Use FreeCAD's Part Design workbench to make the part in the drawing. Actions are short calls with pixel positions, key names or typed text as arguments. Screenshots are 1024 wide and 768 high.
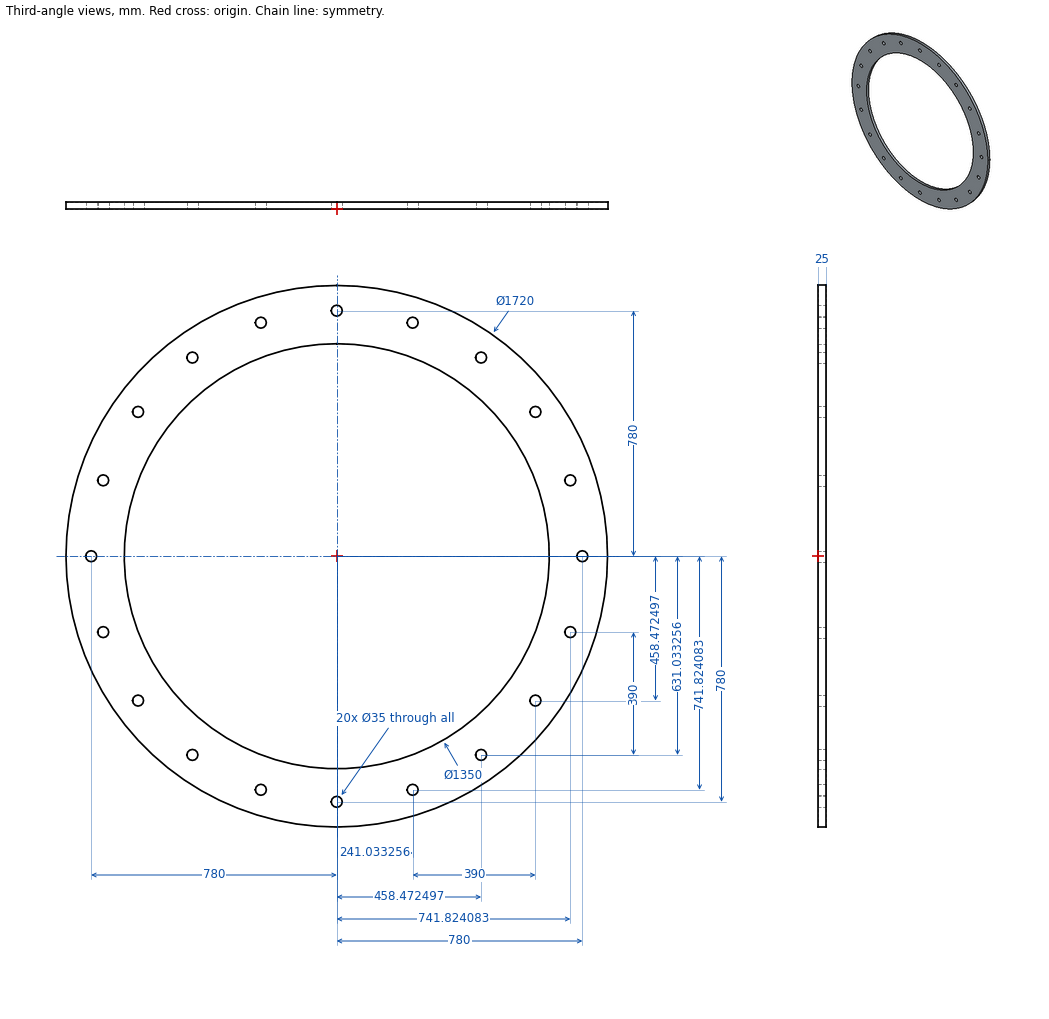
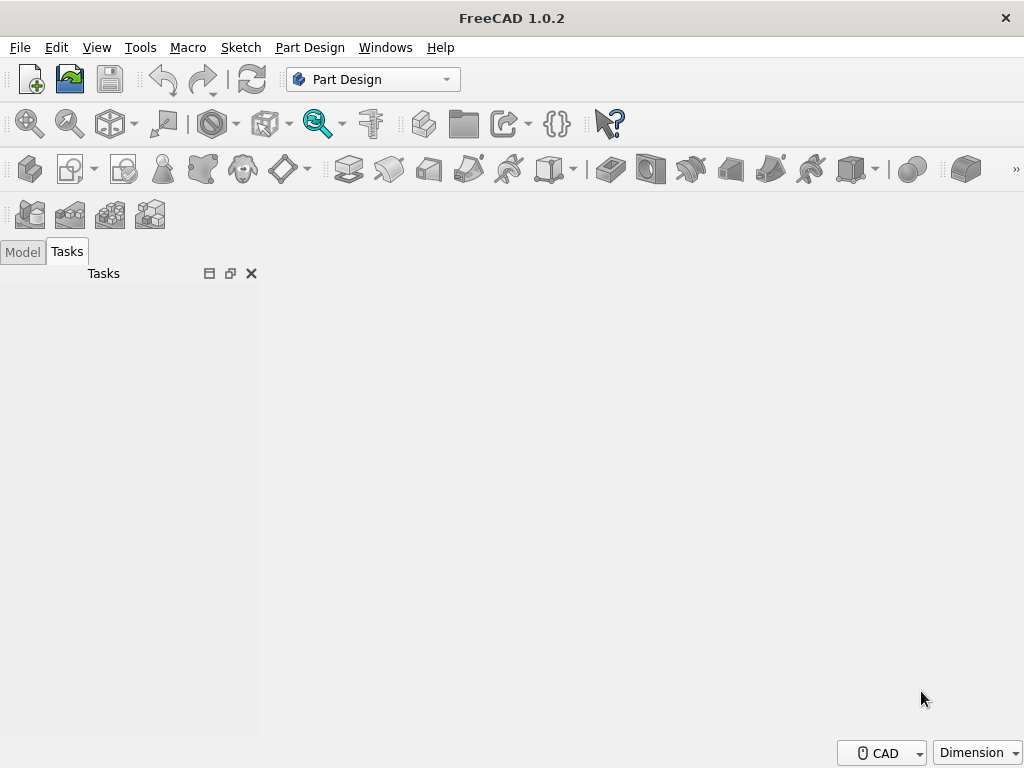
key(ctrl+n)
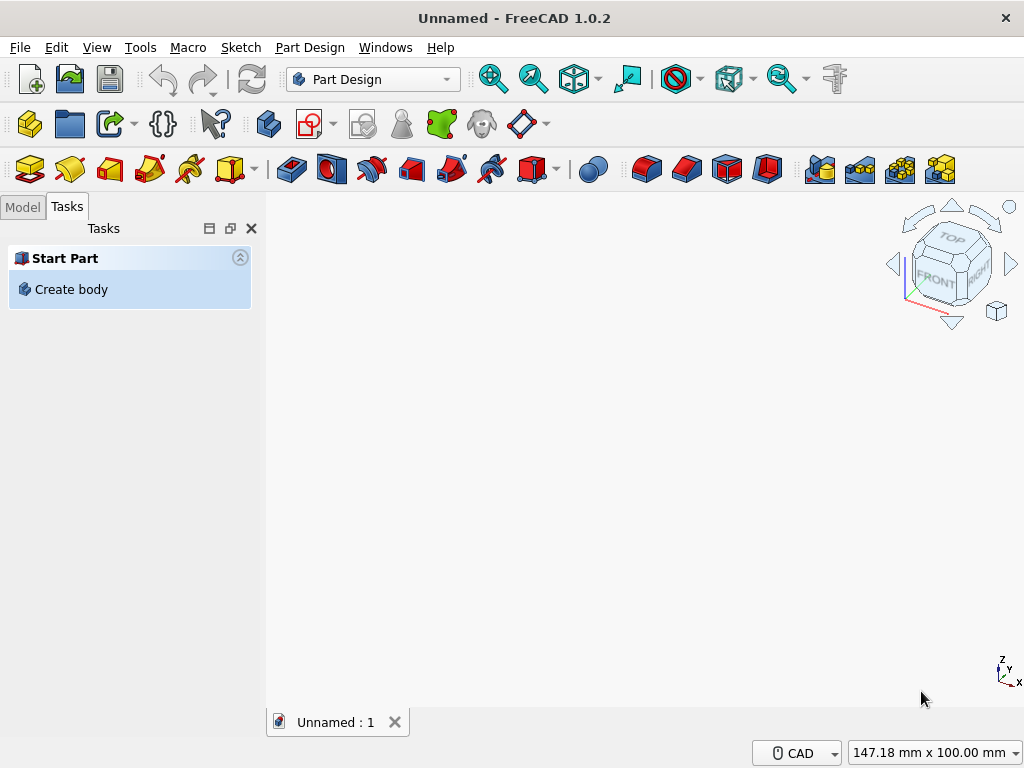
click(310, 124)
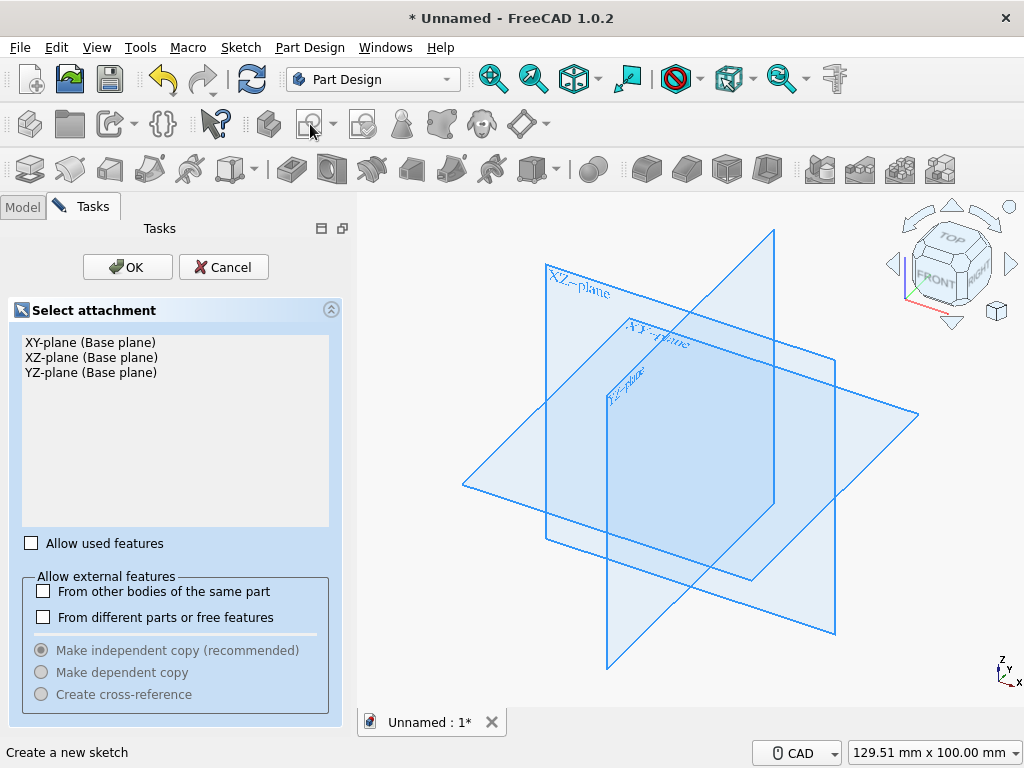
click(82, 358)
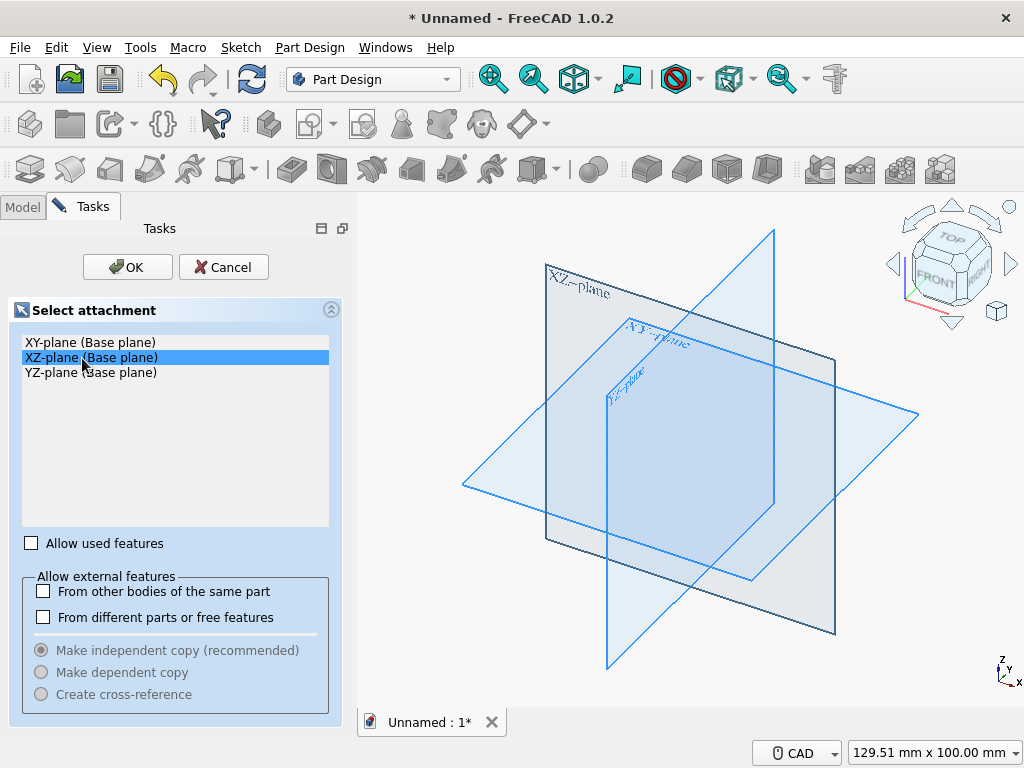
click(128, 267)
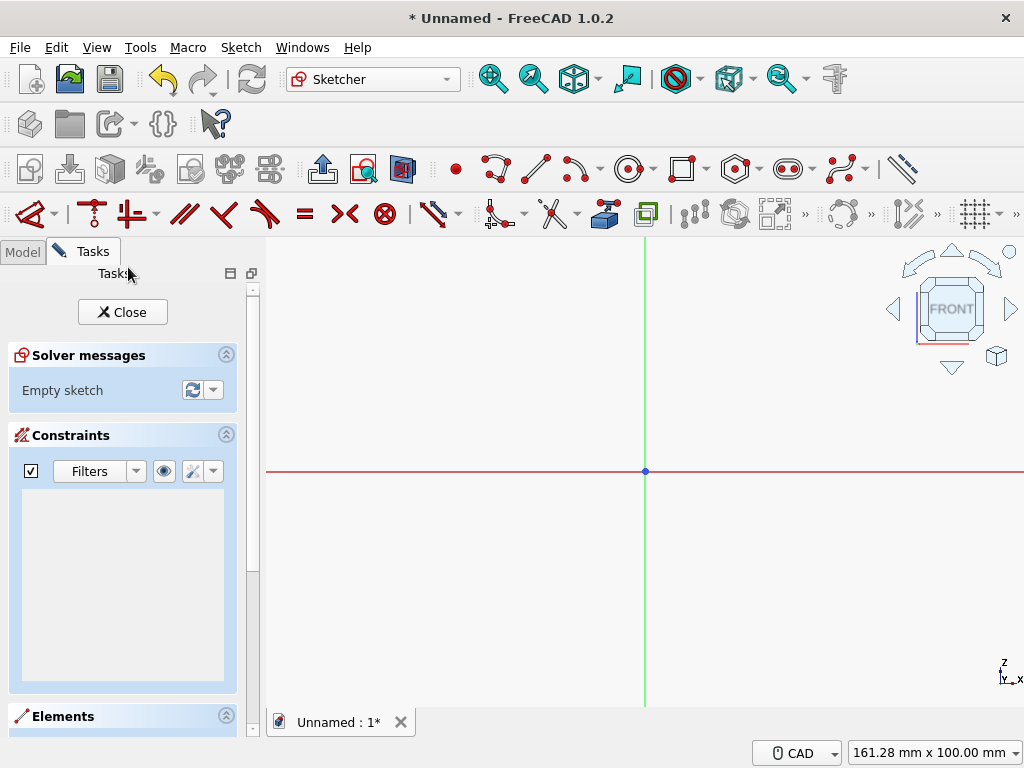
scroll(574, 472, down, 16)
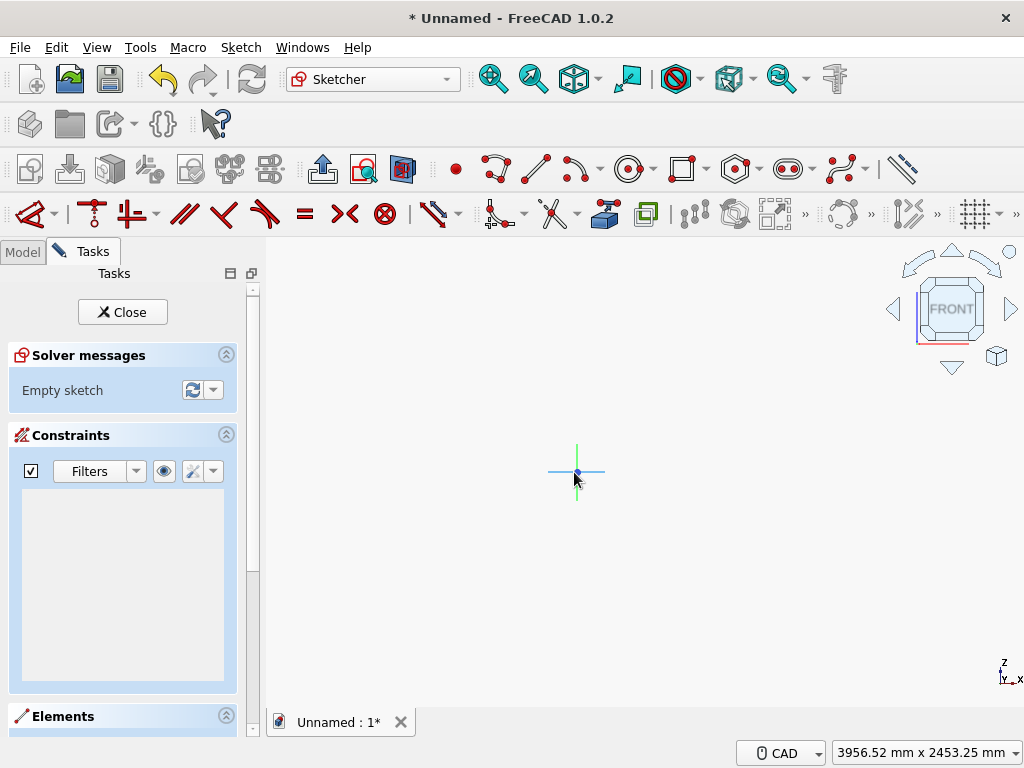
key(g)
key(c)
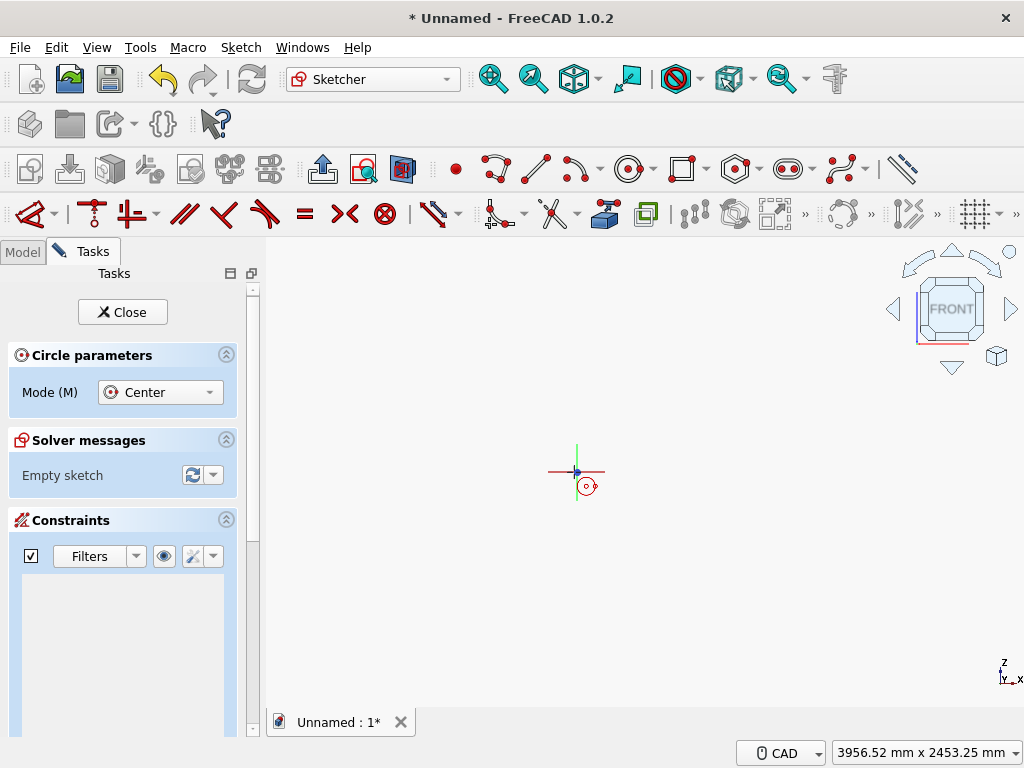
click(577, 472)
move(694, 356)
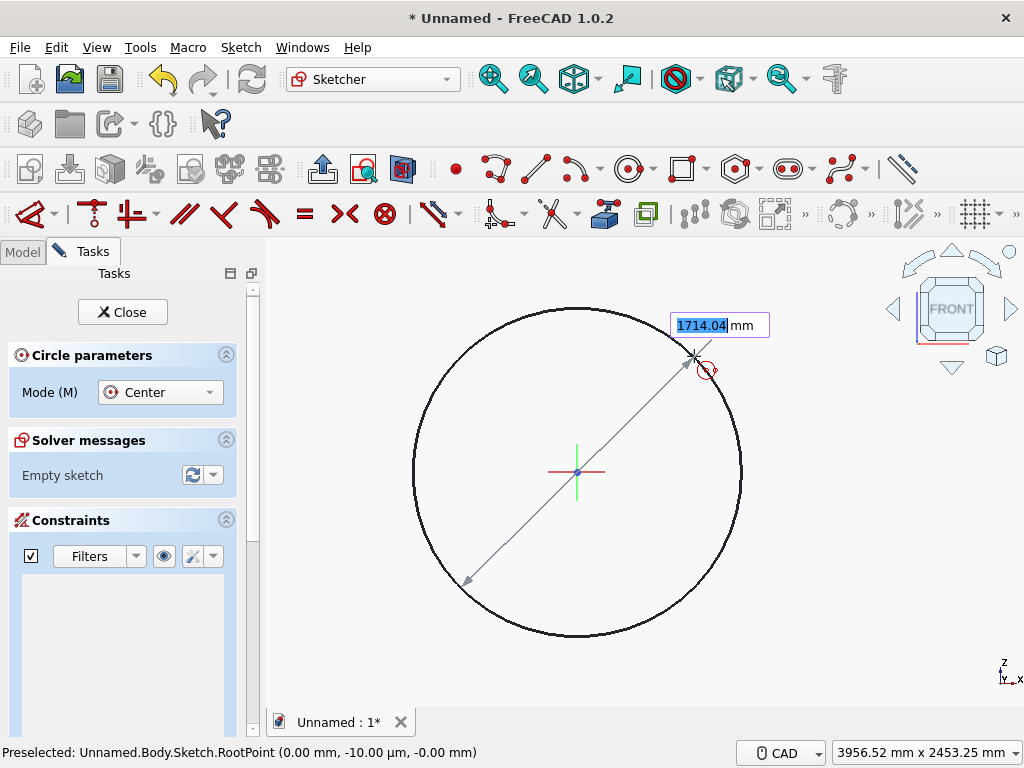
text(1720)
key(Return)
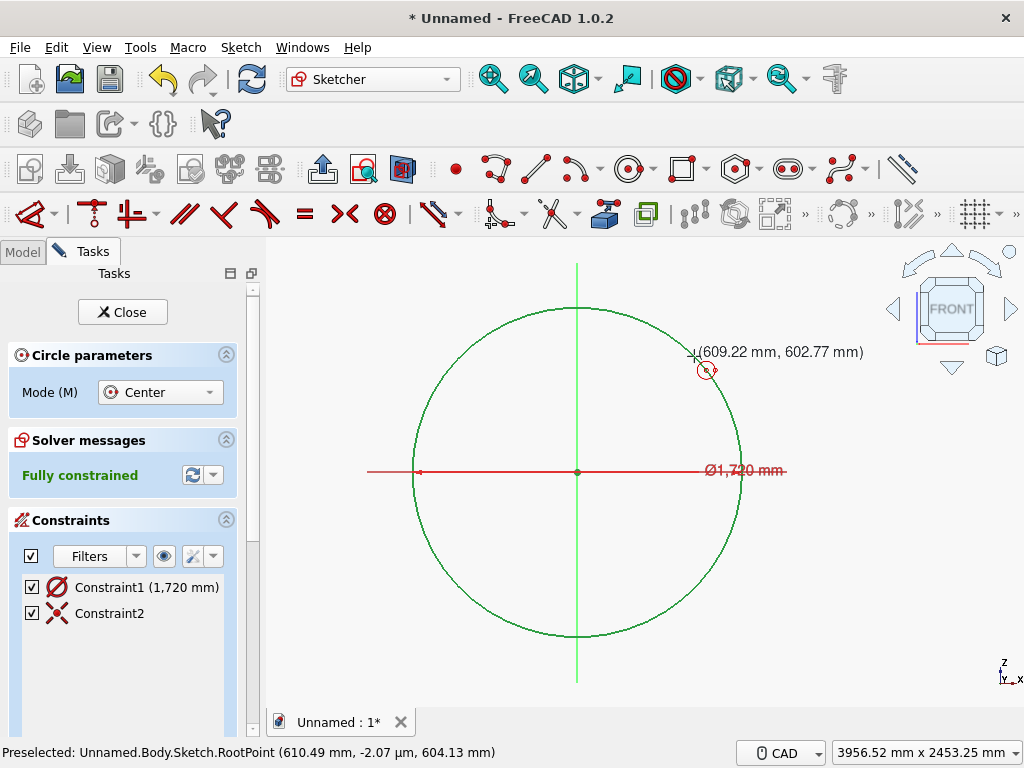
click(577, 472)
move(669, 381)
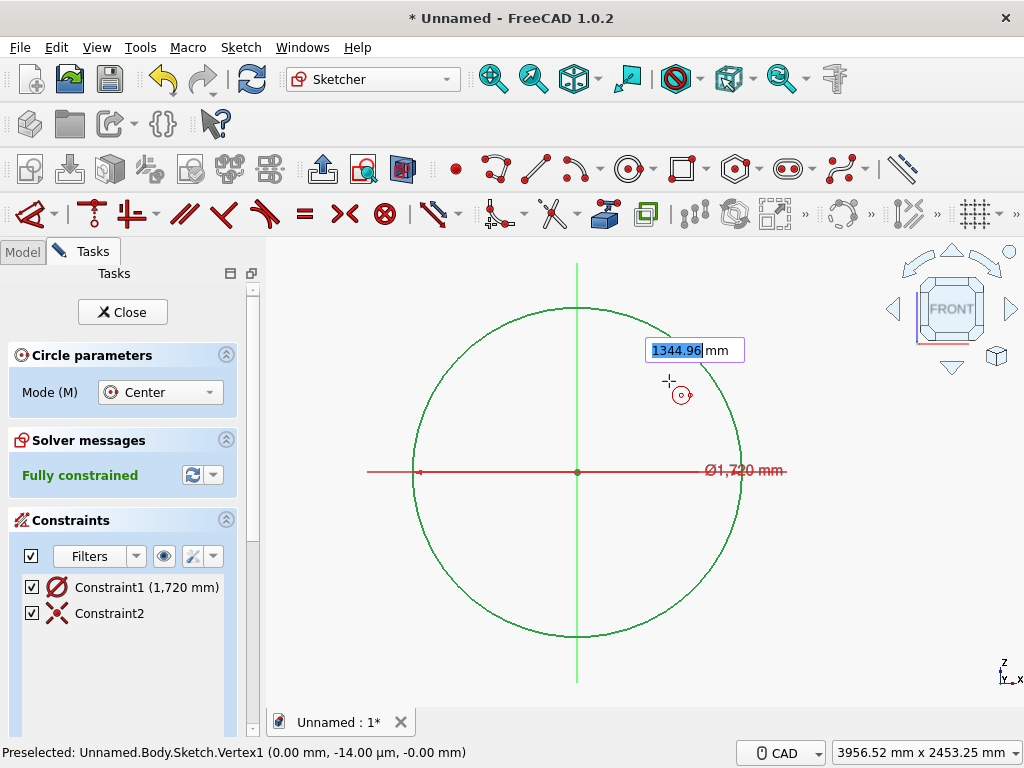
text(1350)
key(Return)
key(Escape)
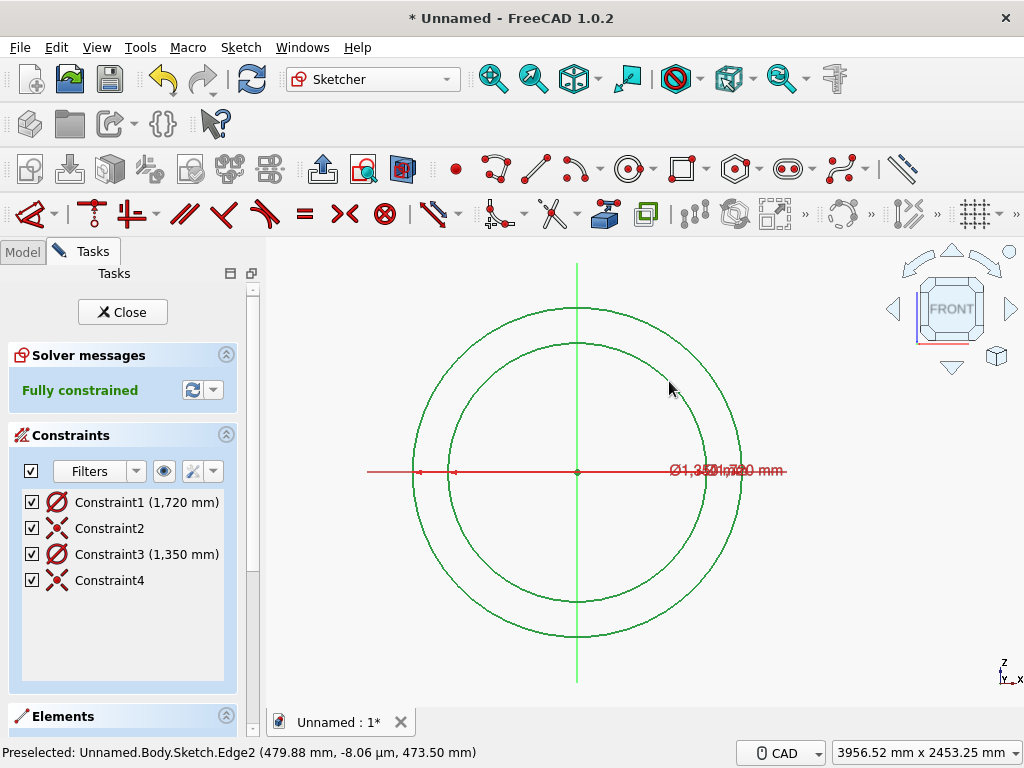
click(123, 312)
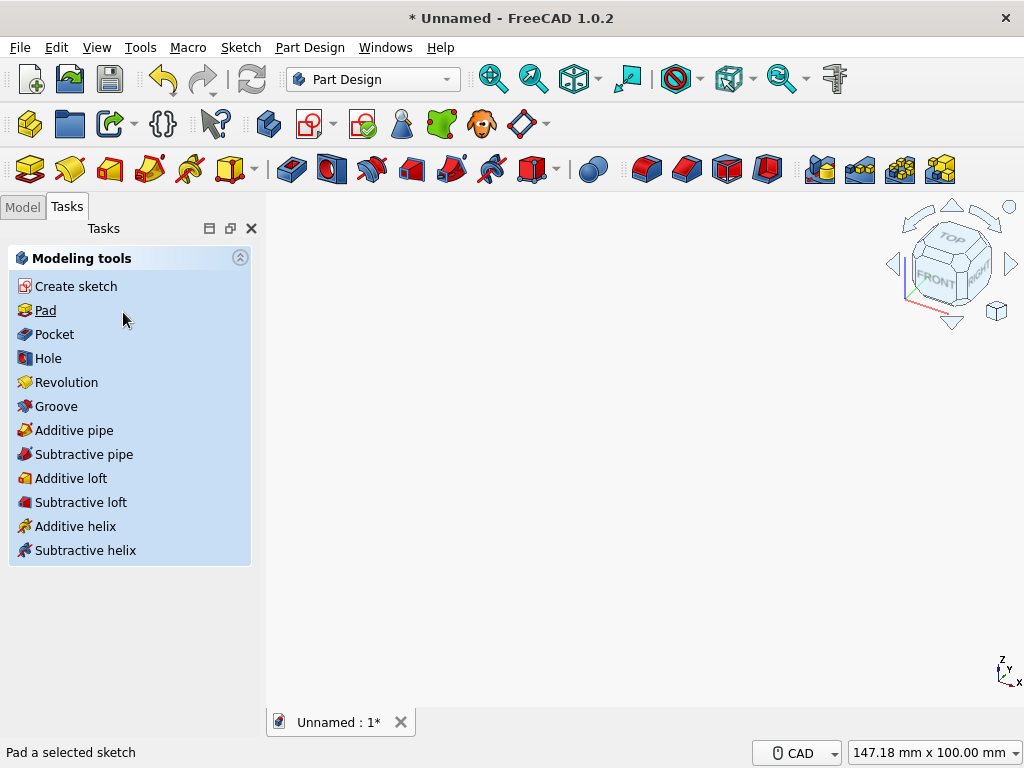
click(30, 170)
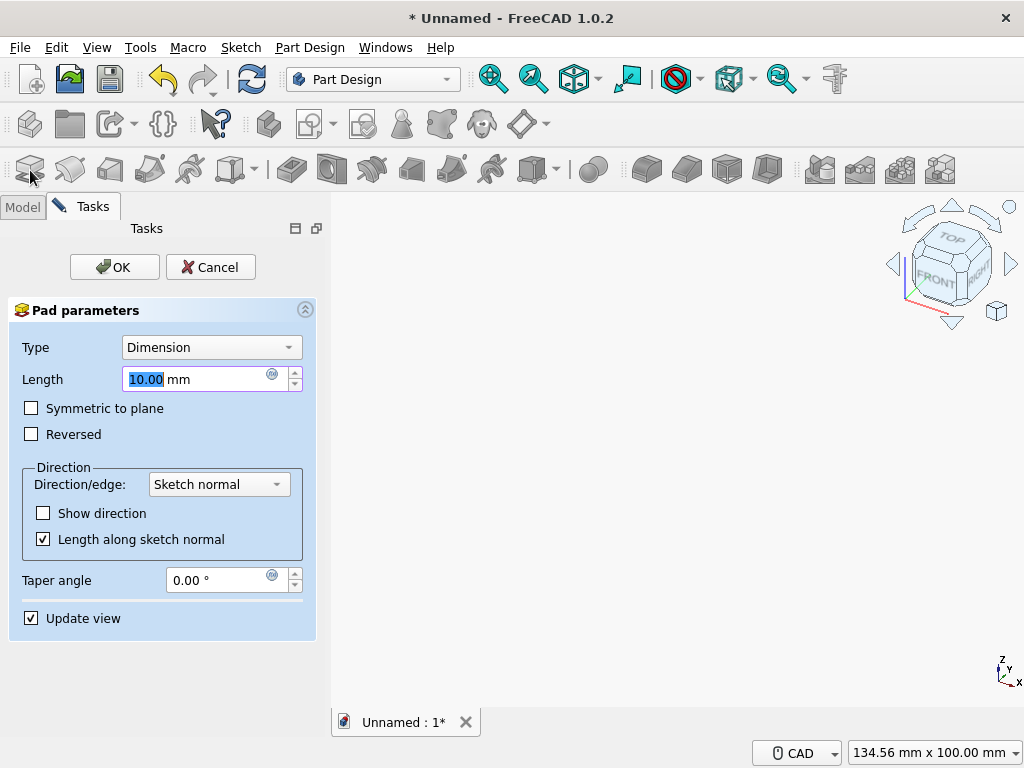
text(25)
key(Tab)